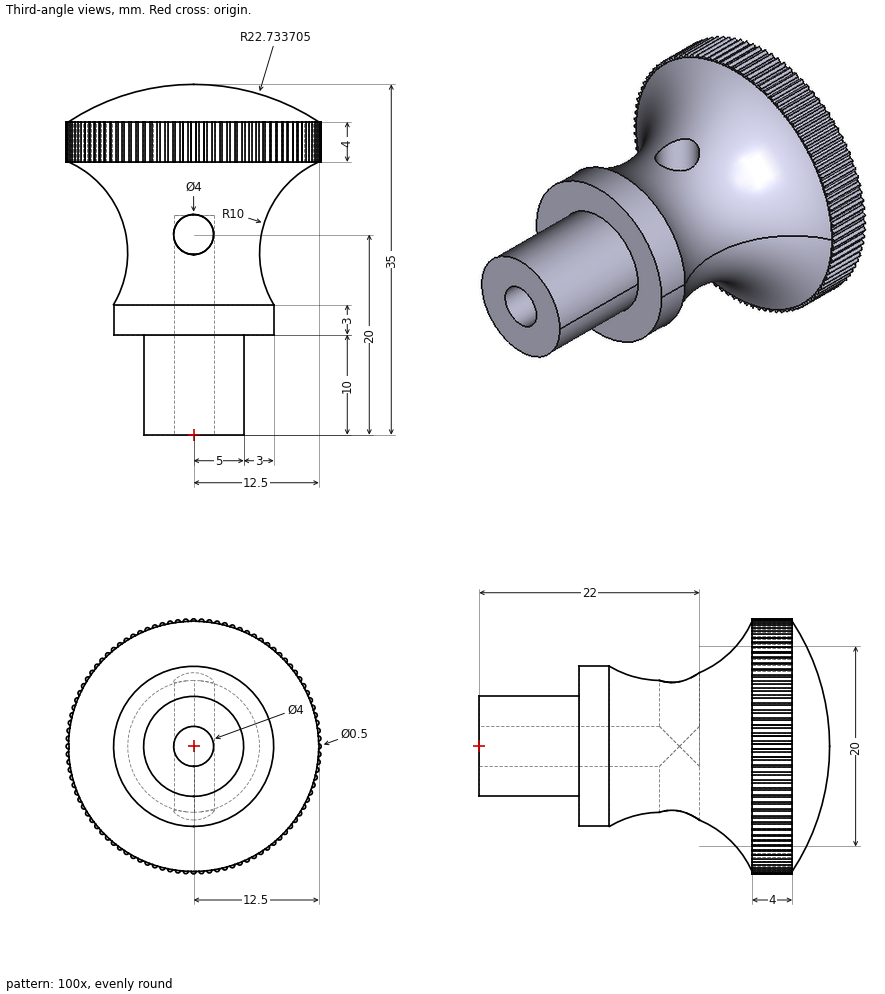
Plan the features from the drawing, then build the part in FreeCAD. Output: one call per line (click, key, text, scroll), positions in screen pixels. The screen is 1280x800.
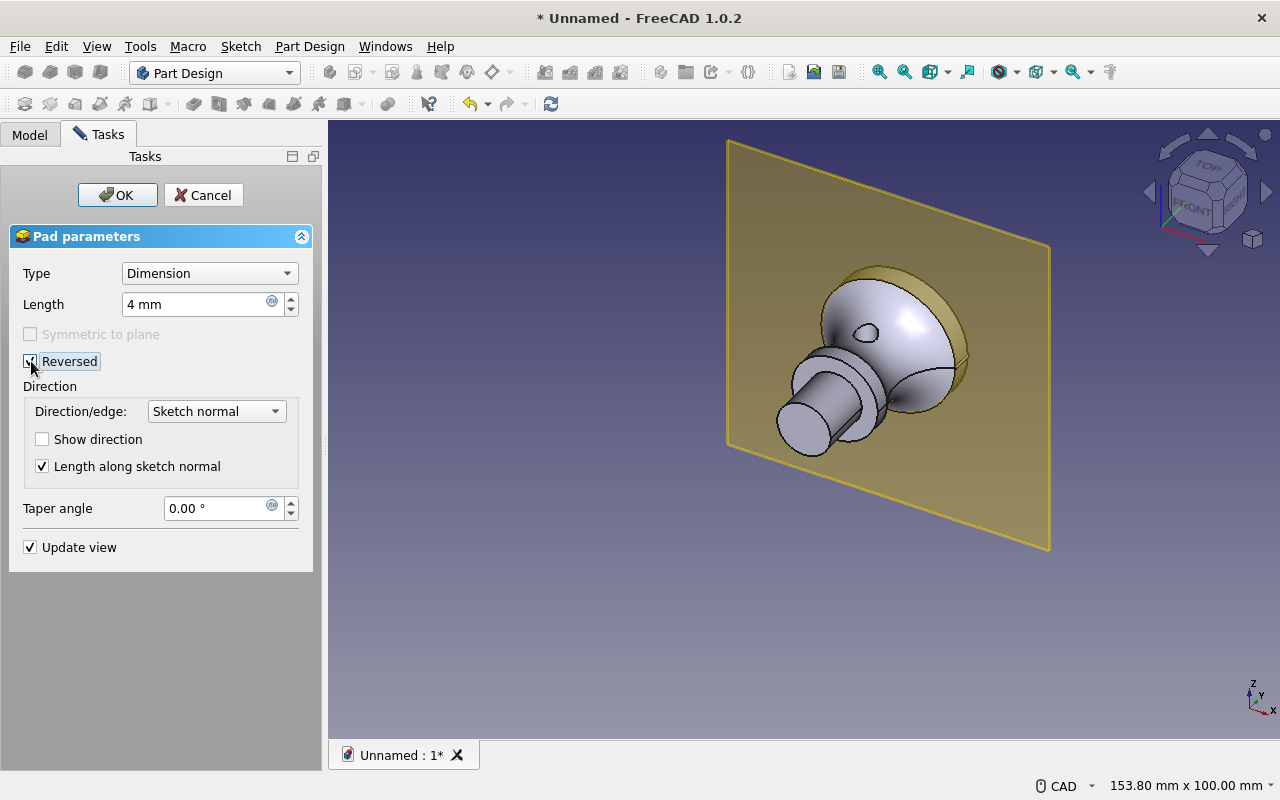
click(118, 195)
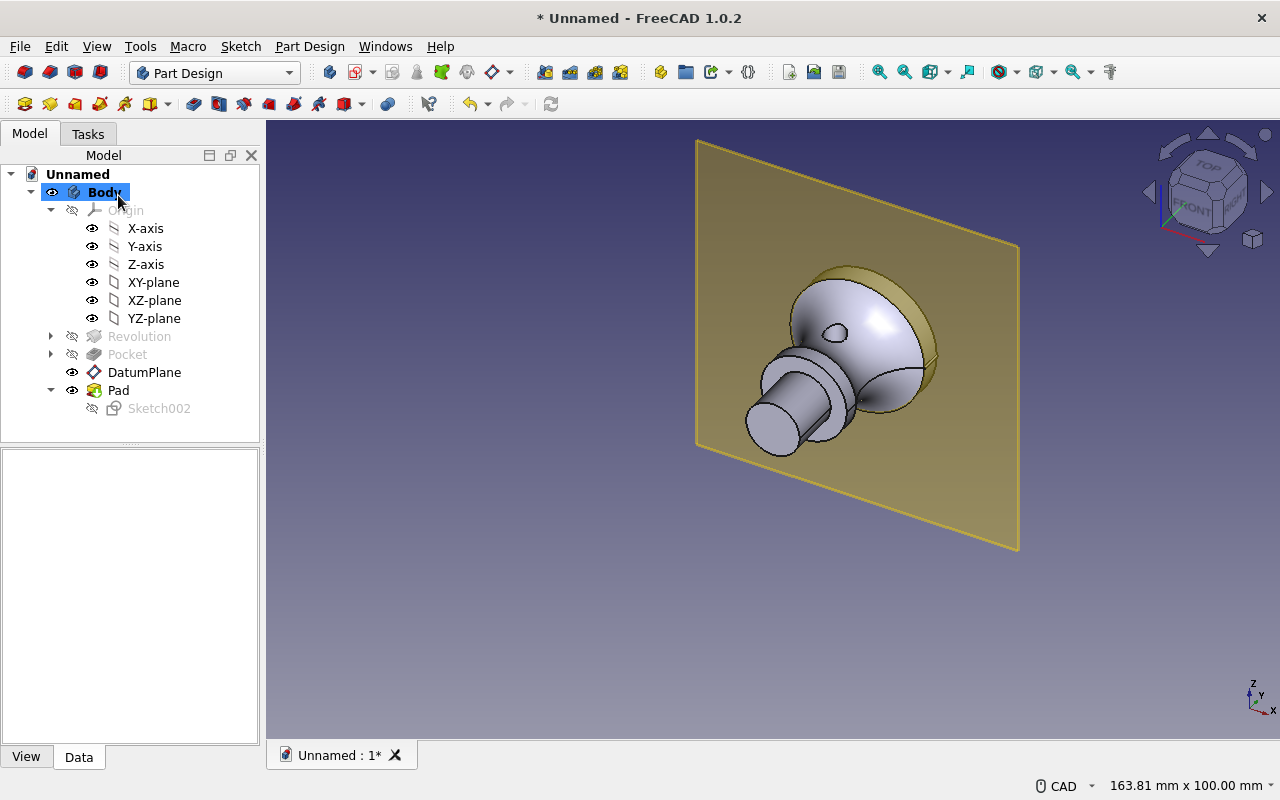
click(117, 372)
key(space)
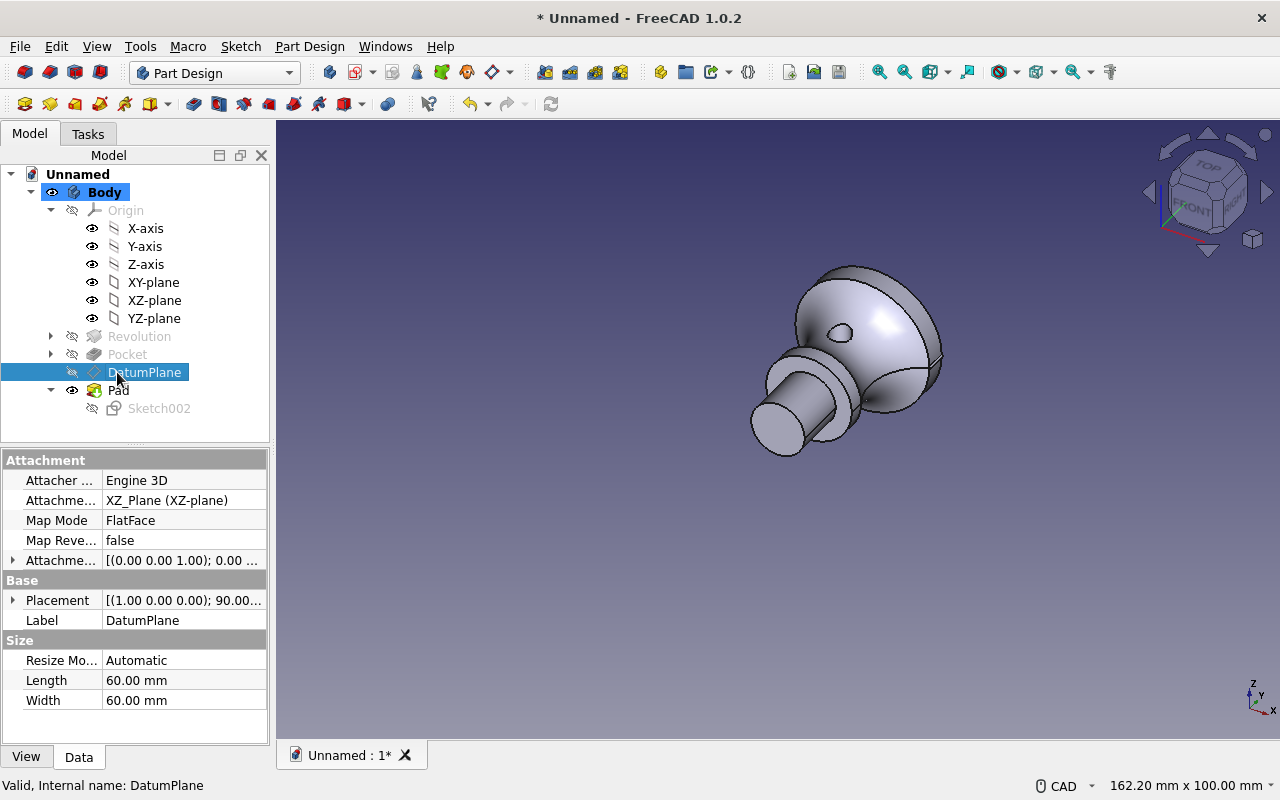
click(117, 390)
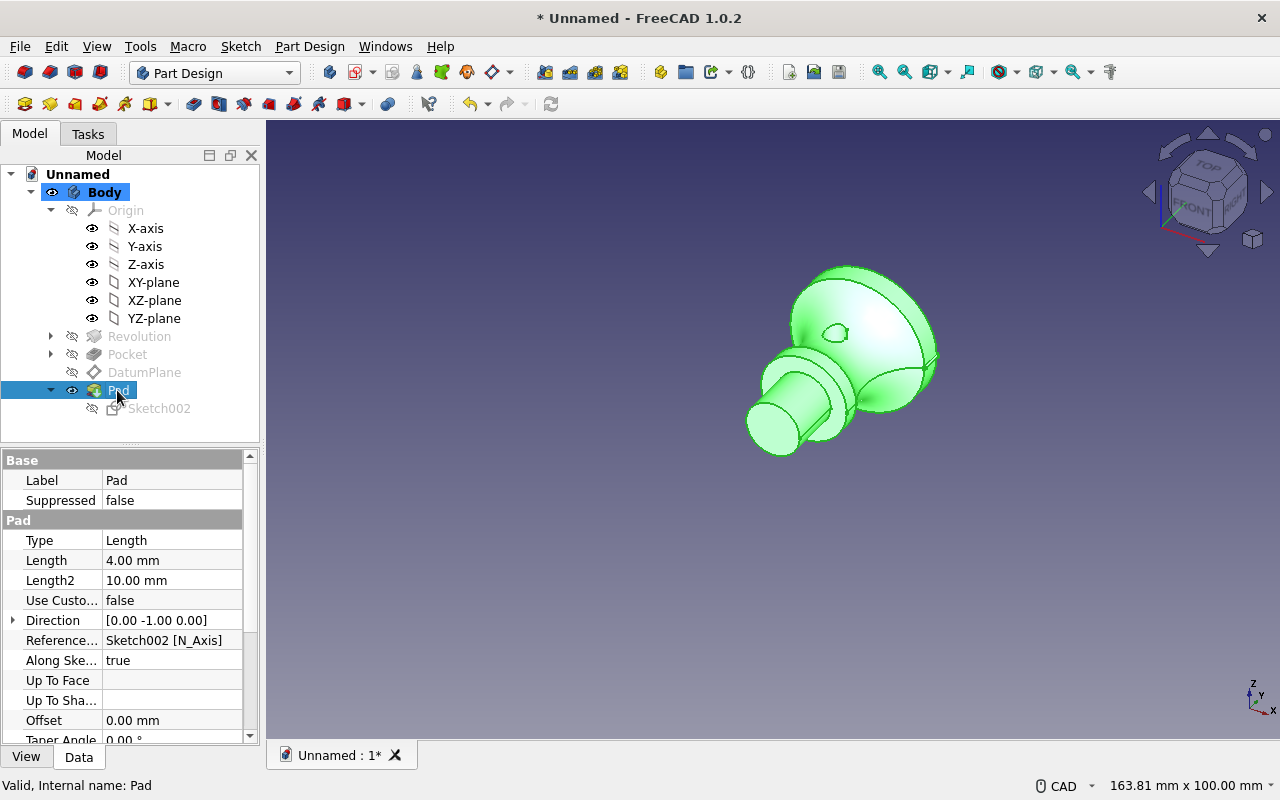
click(595, 72)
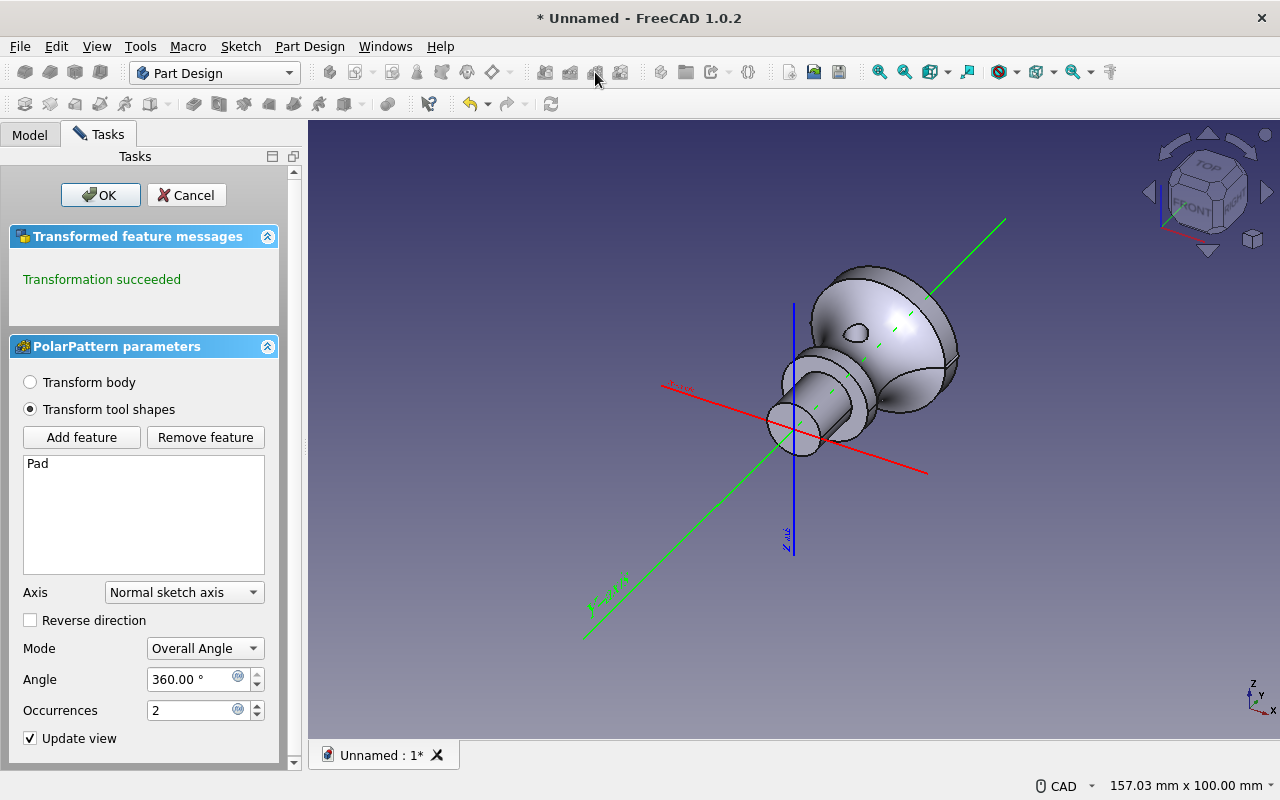
click(185, 592)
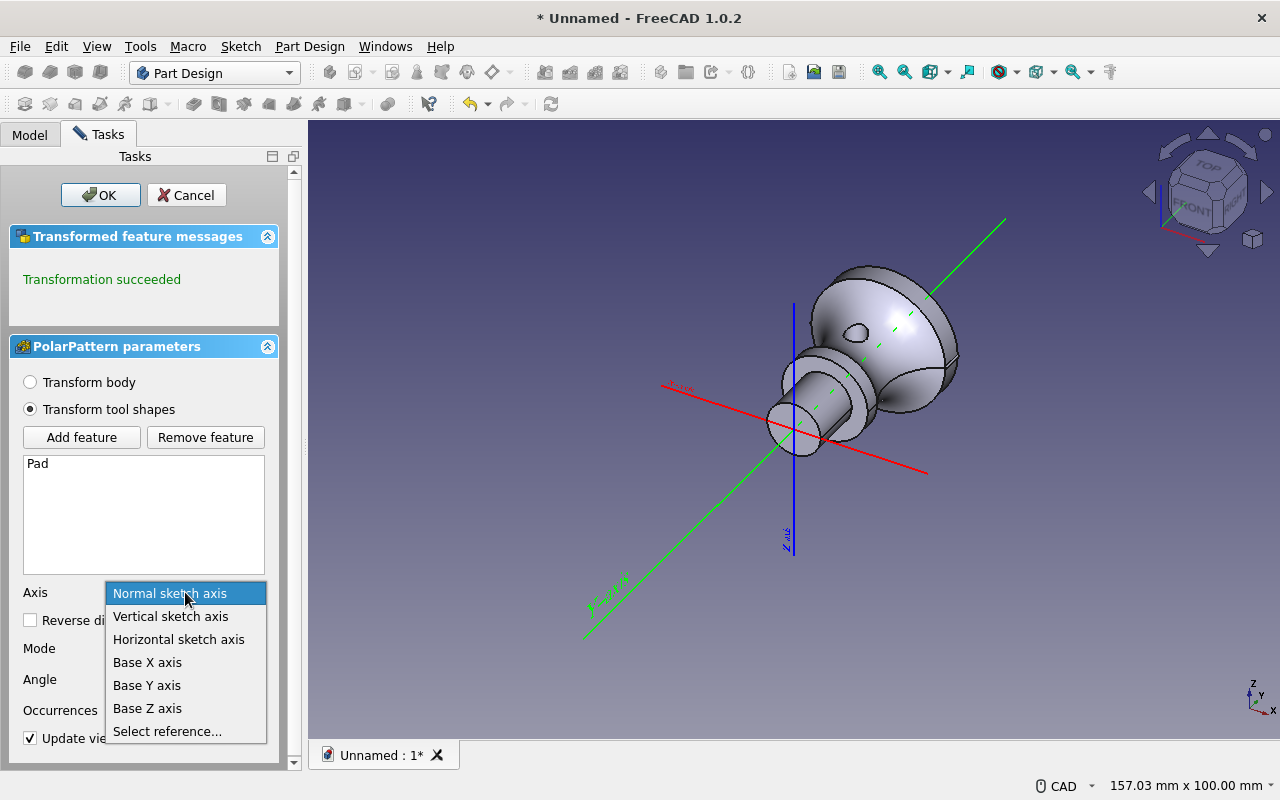
click(184, 686)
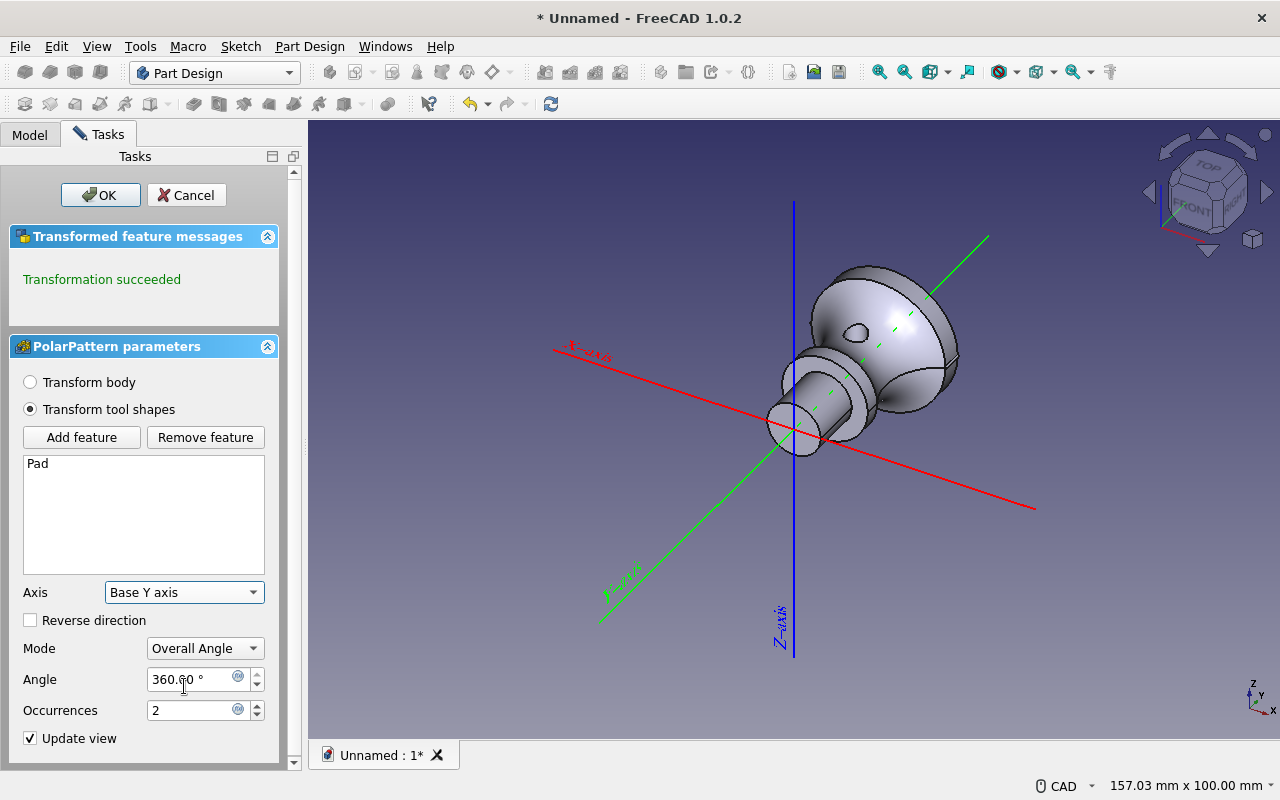
triple_click(199, 710)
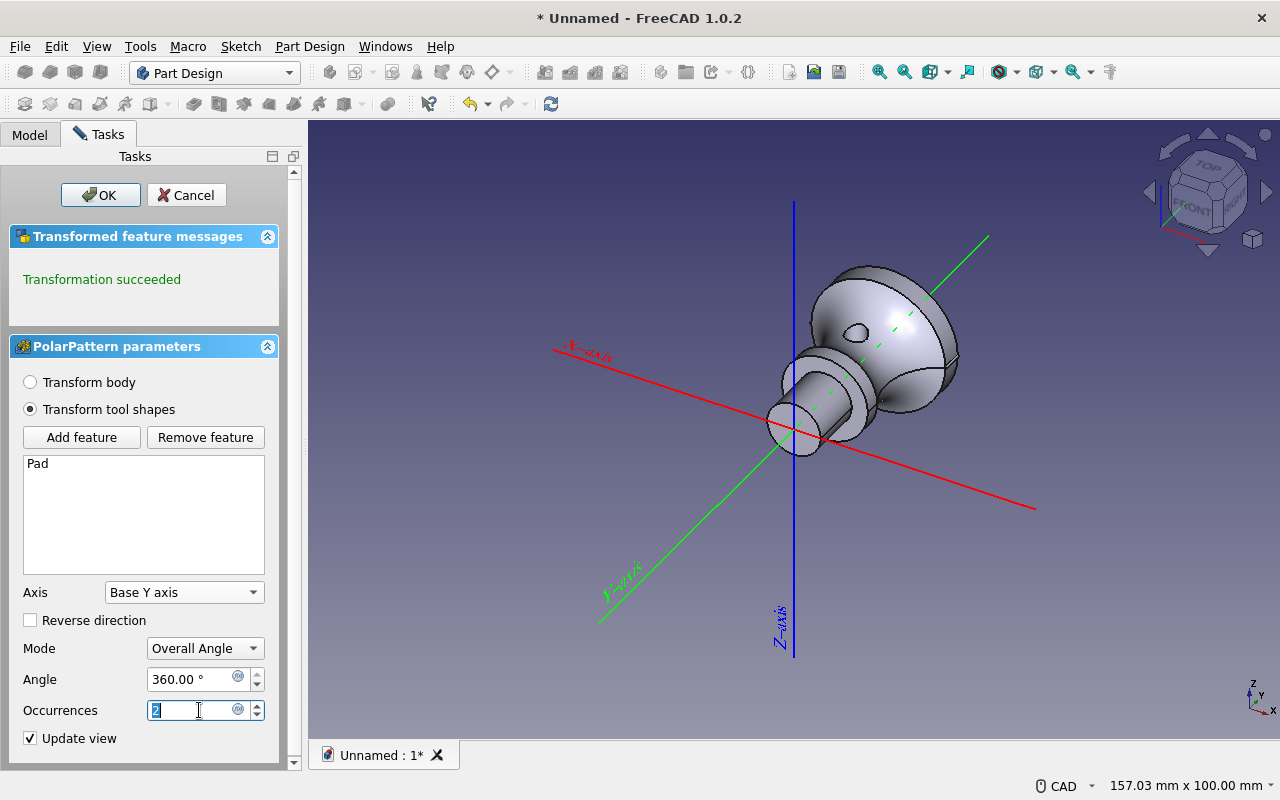
text(100)
key(Tab)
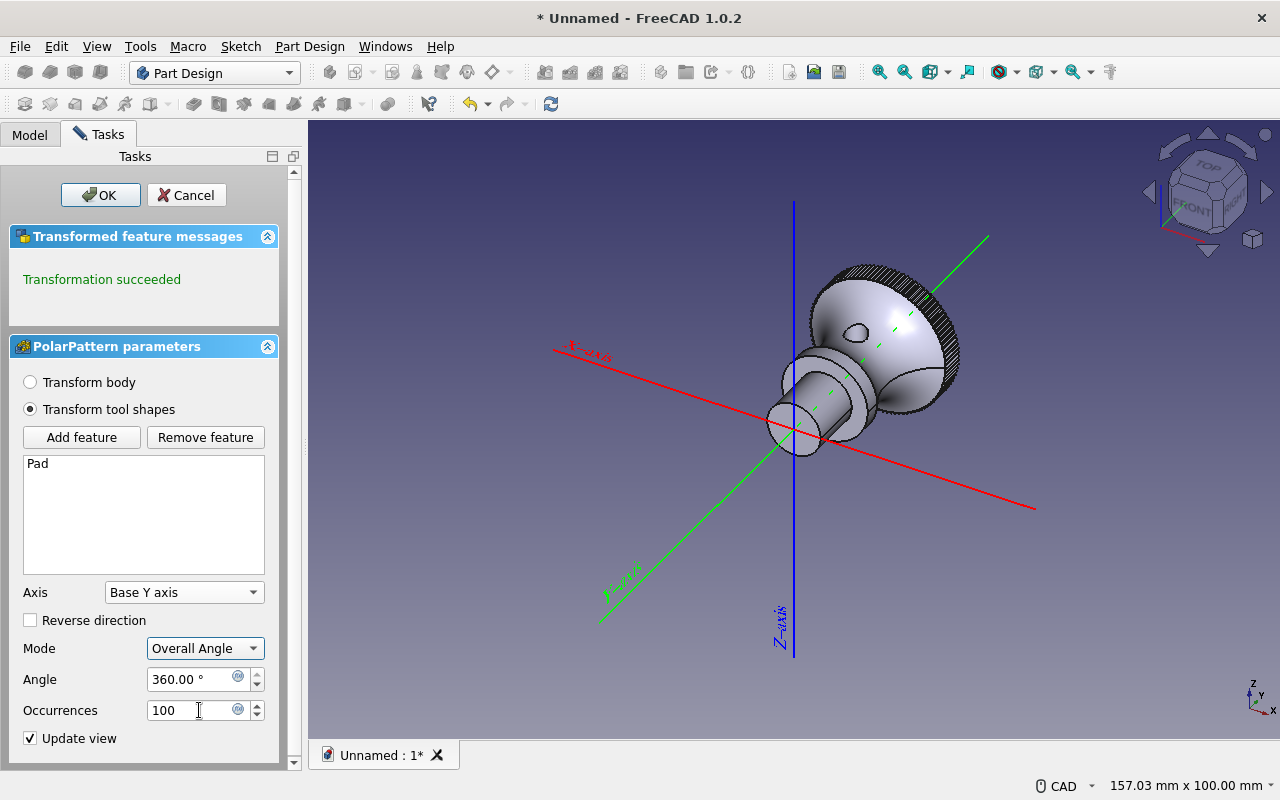
click(101, 195)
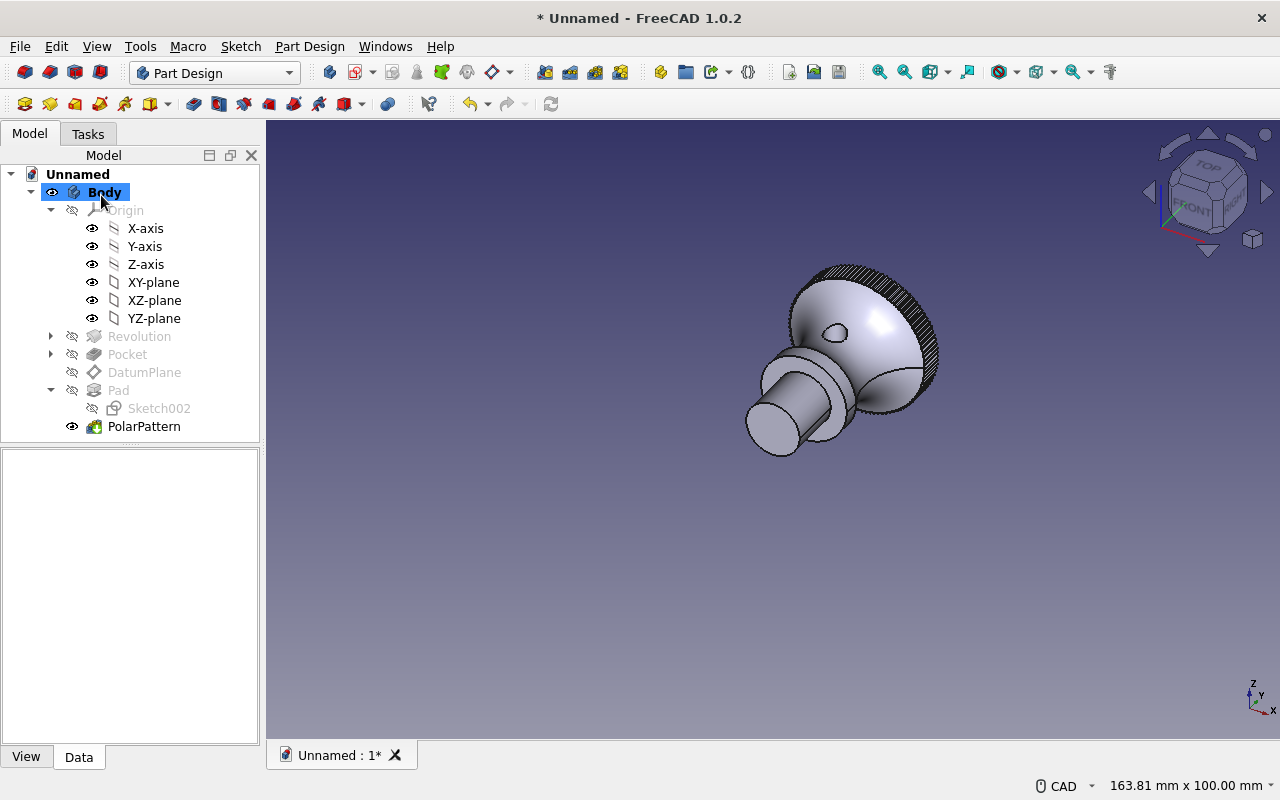
click(354, 72)